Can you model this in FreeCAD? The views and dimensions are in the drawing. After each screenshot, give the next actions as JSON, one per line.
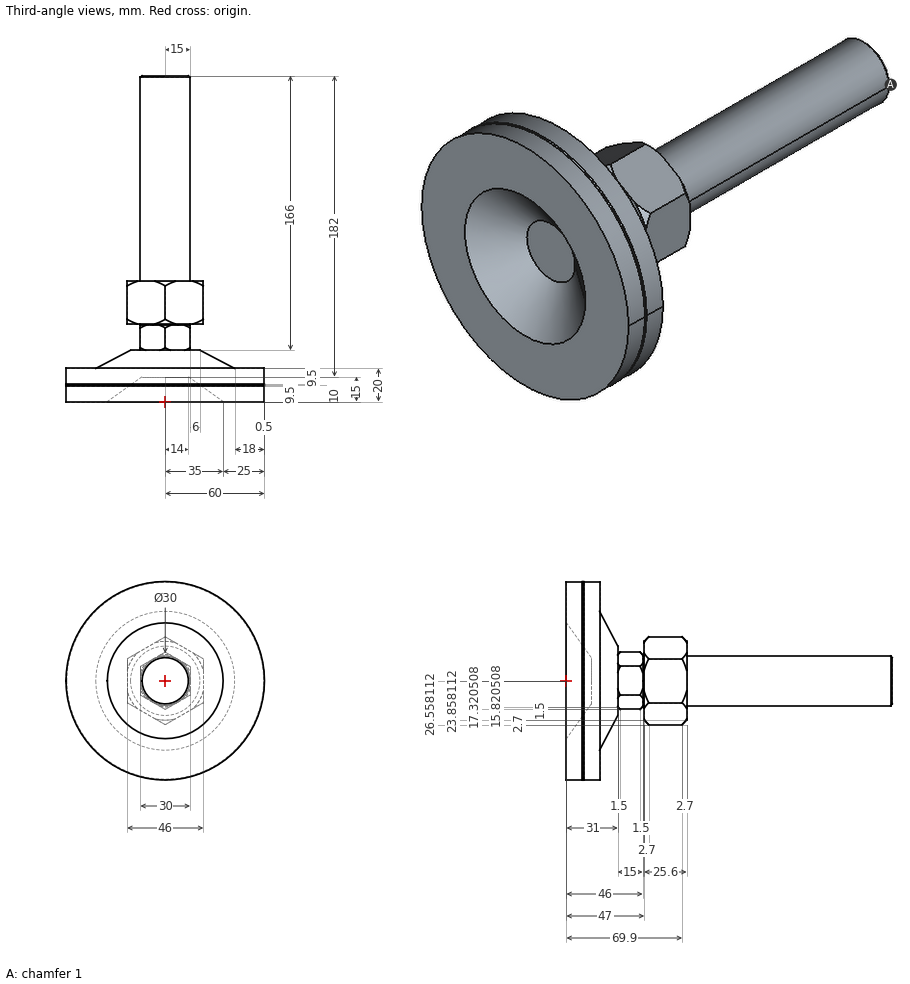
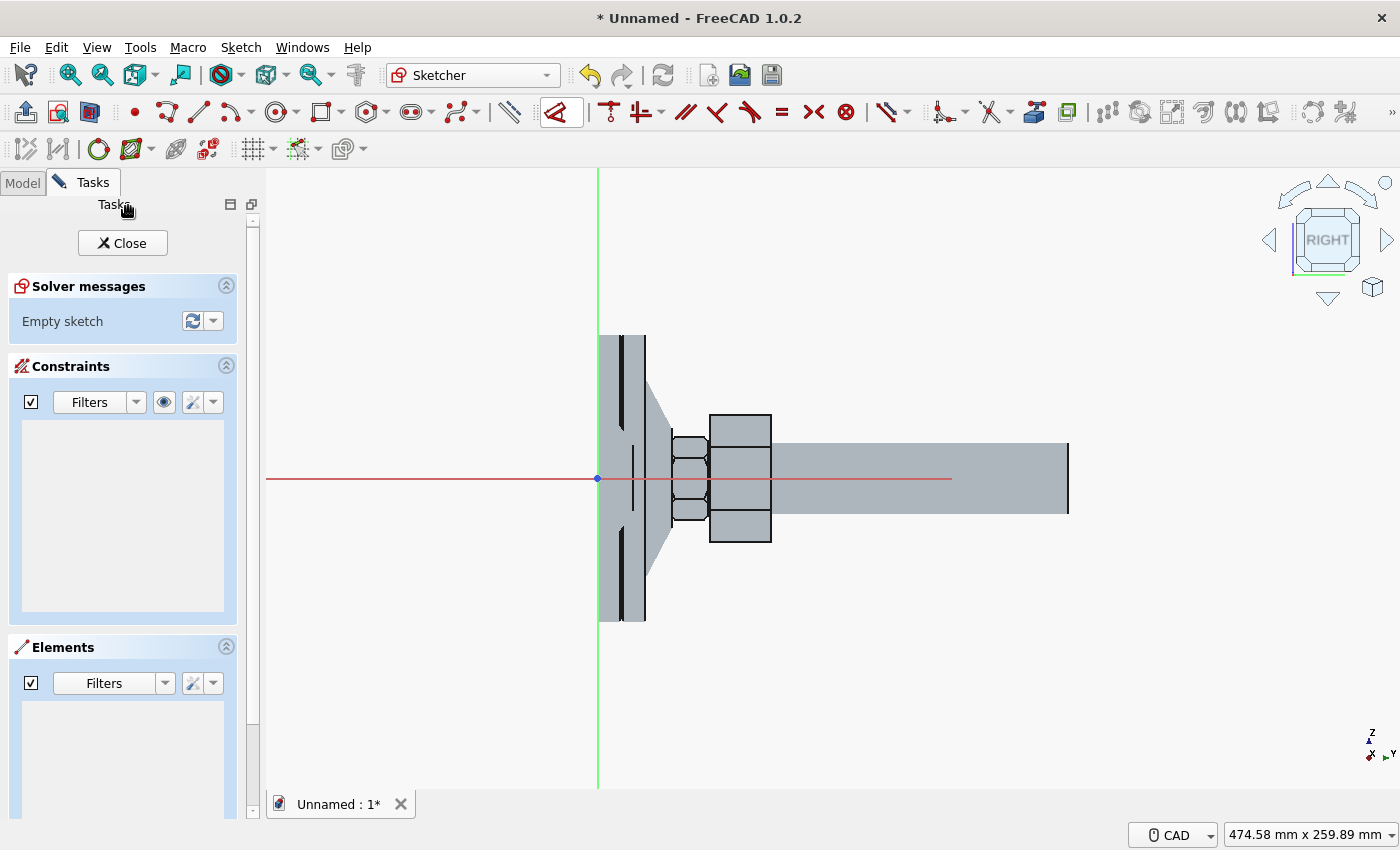
{"action": "scroll", "coordinate": [738, 545], "scroll_direction": "up", "scroll_amount": 12}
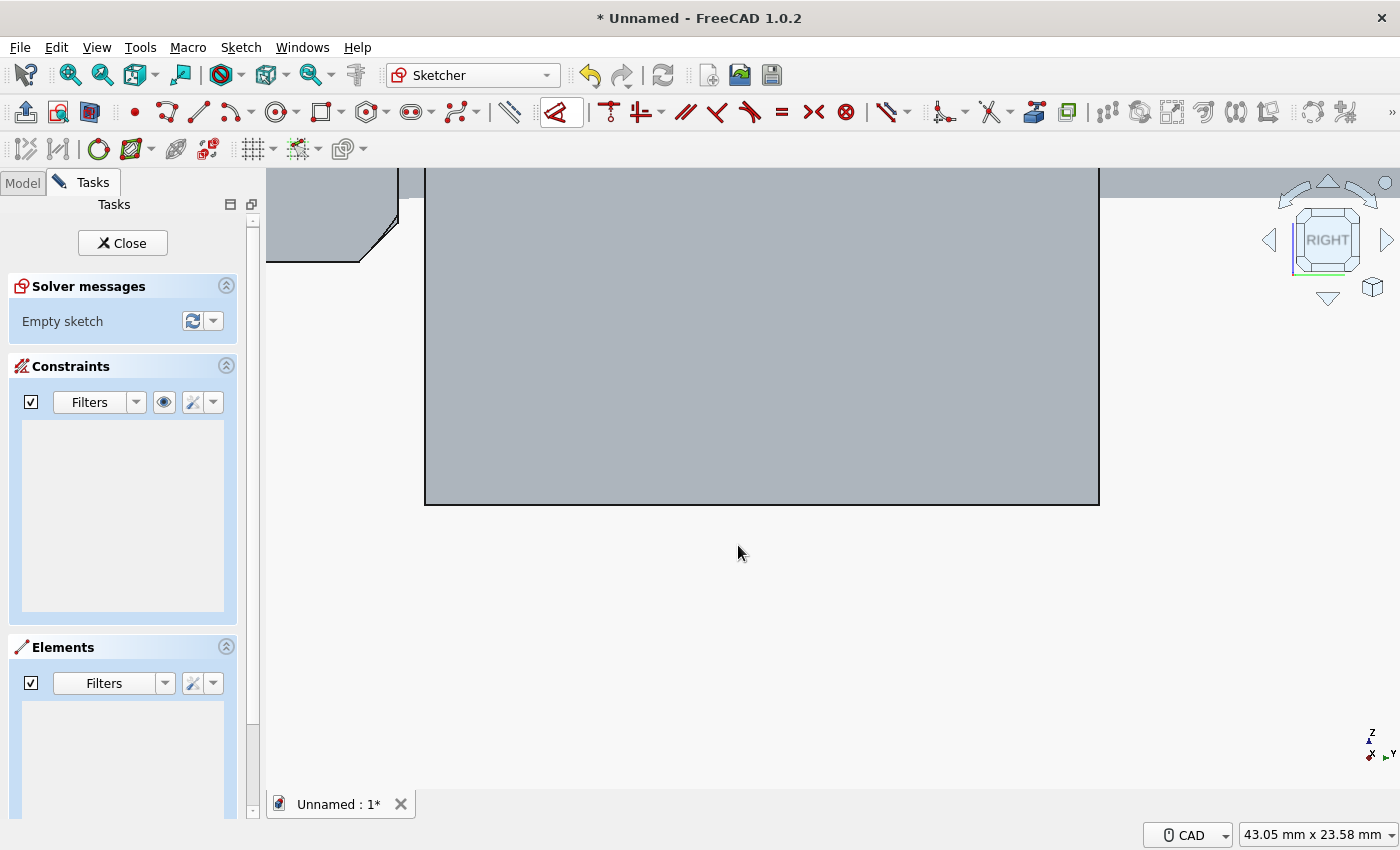
{"action": "key", "text": "g m"}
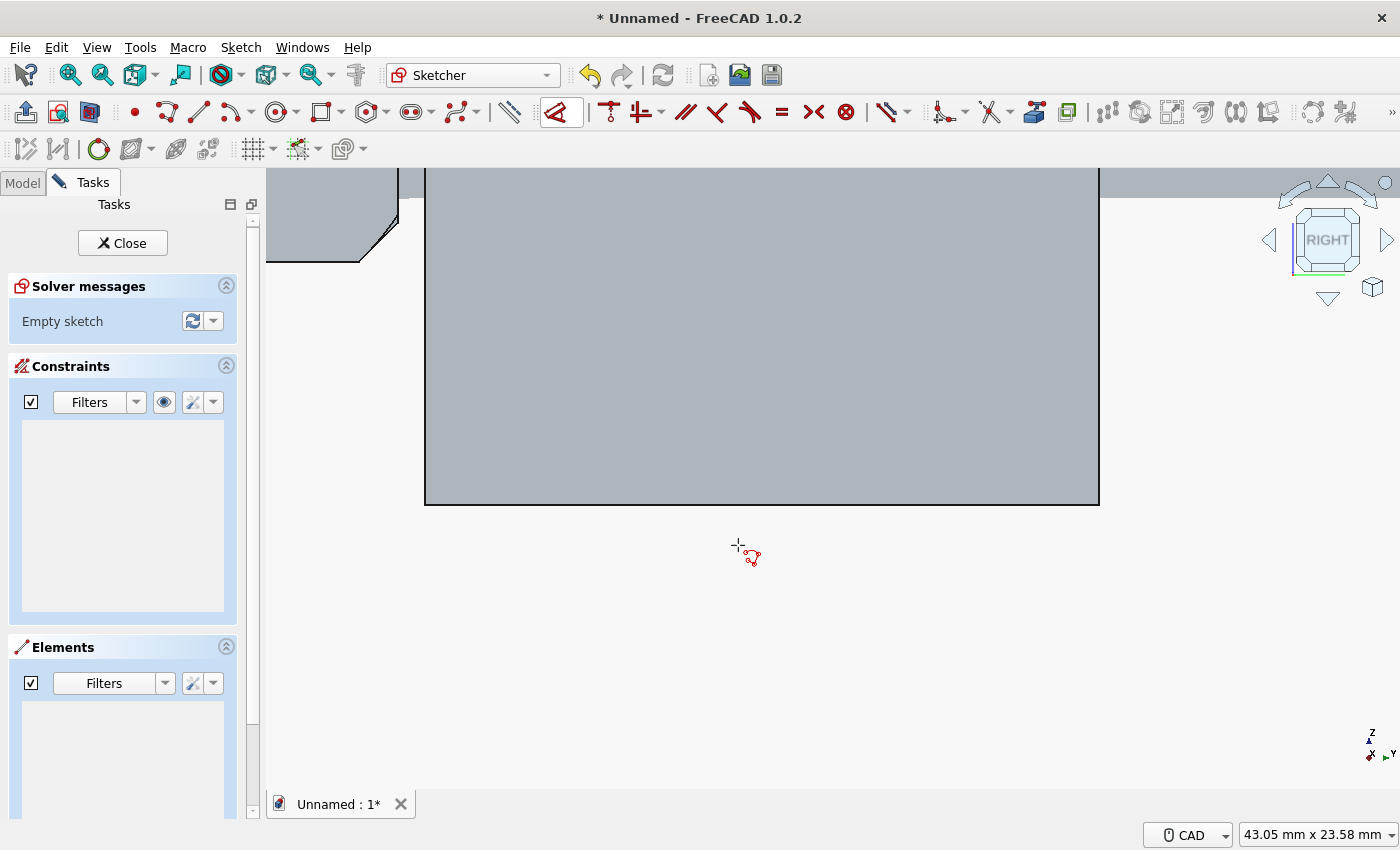
{"action": "left_click", "coordinate": [1028, 505]}
{"action": "left_click", "coordinate": [1099, 505]}
{"action": "left_click", "coordinate": [1099, 434]}
{"action": "left_click", "coordinate": [1028, 506]}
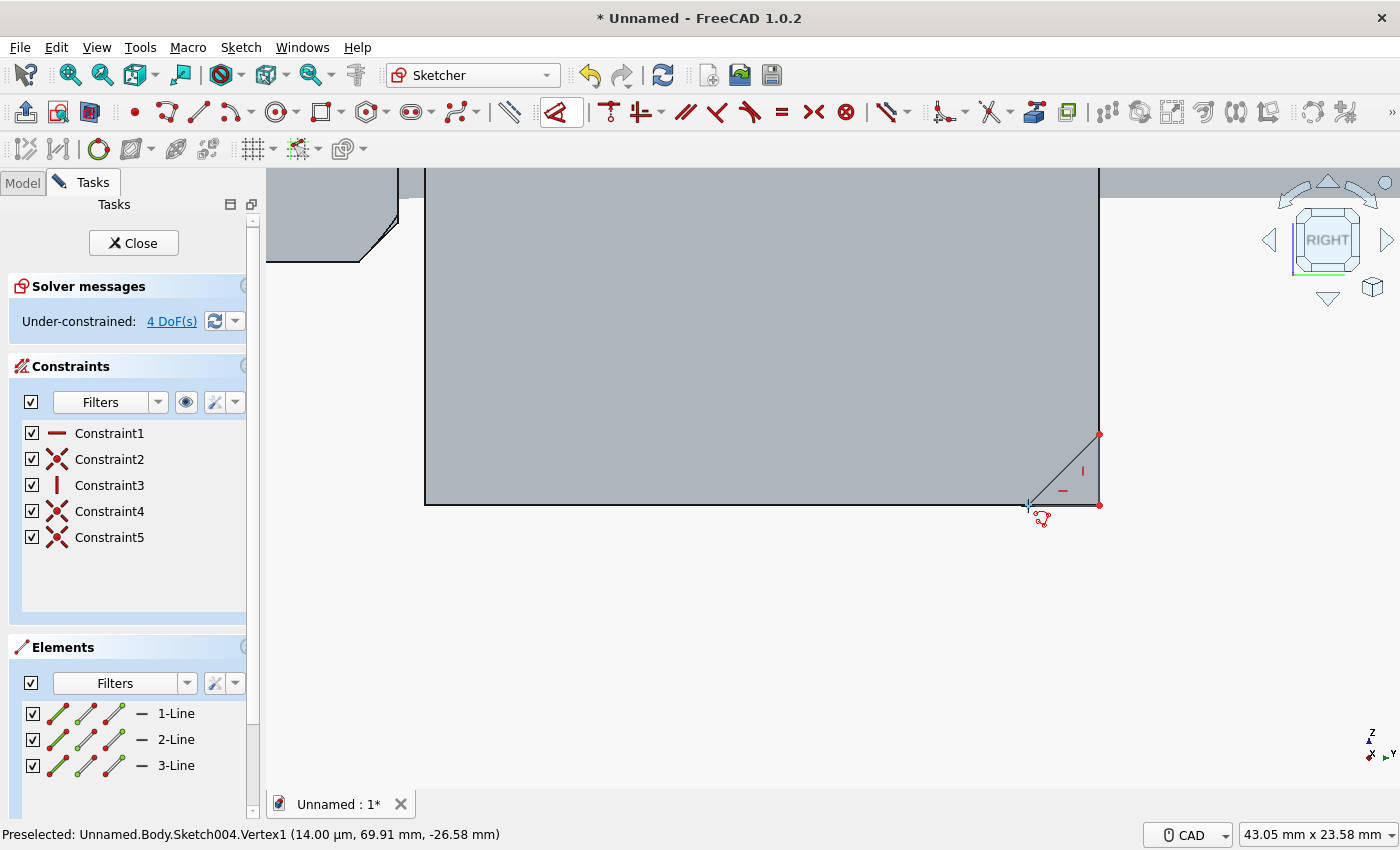
{"action": "left_click", "coordinate": [425, 434]}
{"action": "left_click", "coordinate": [425, 505]}
{"action": "left_click", "coordinate": [496, 505]}
{"action": "left_click", "coordinate": [425, 435]}
{"action": "key", "text": "Escape"}
{"action": "key", "text": "Escape"}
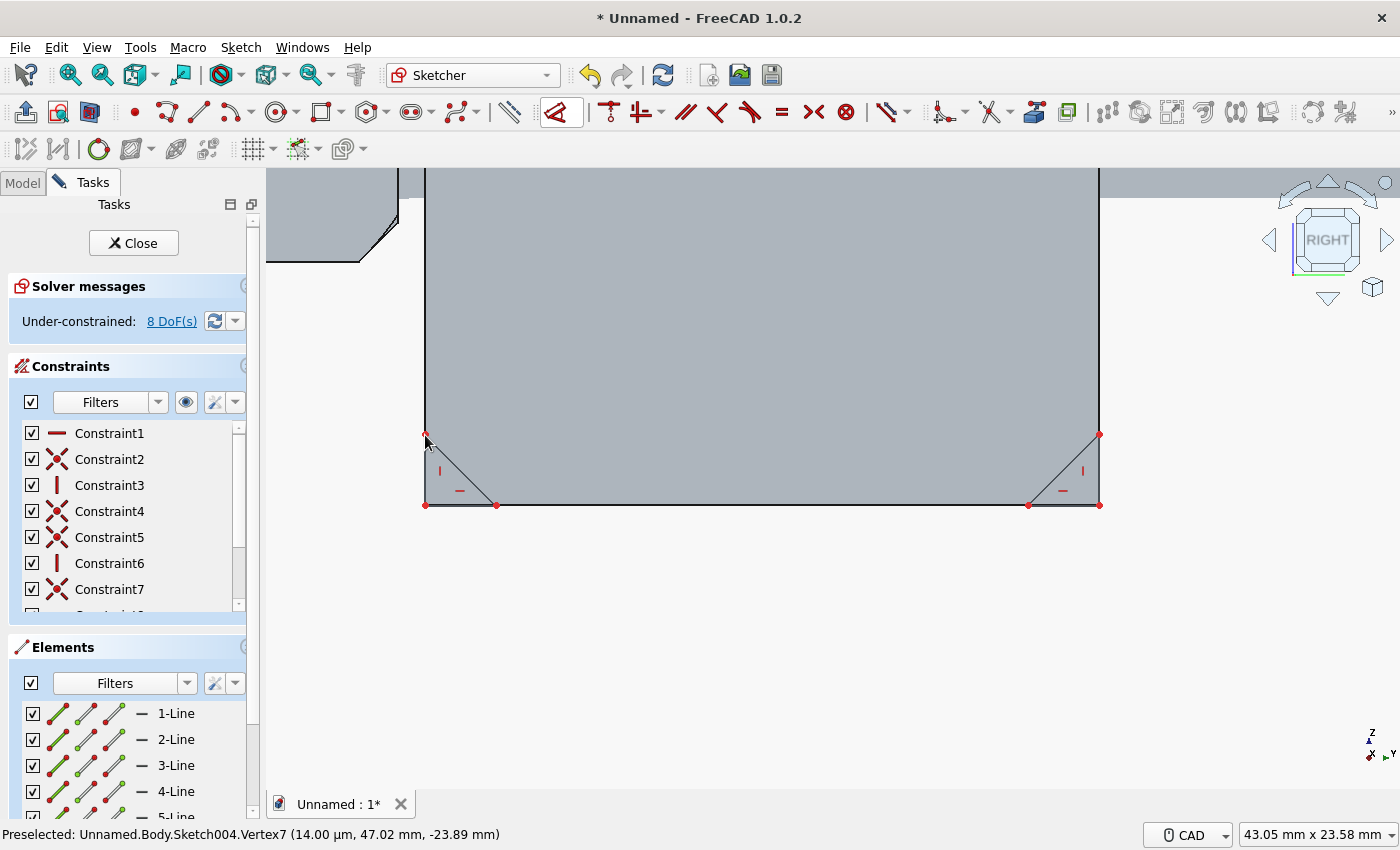
{"action": "left_click", "coordinate": [1049, 506]}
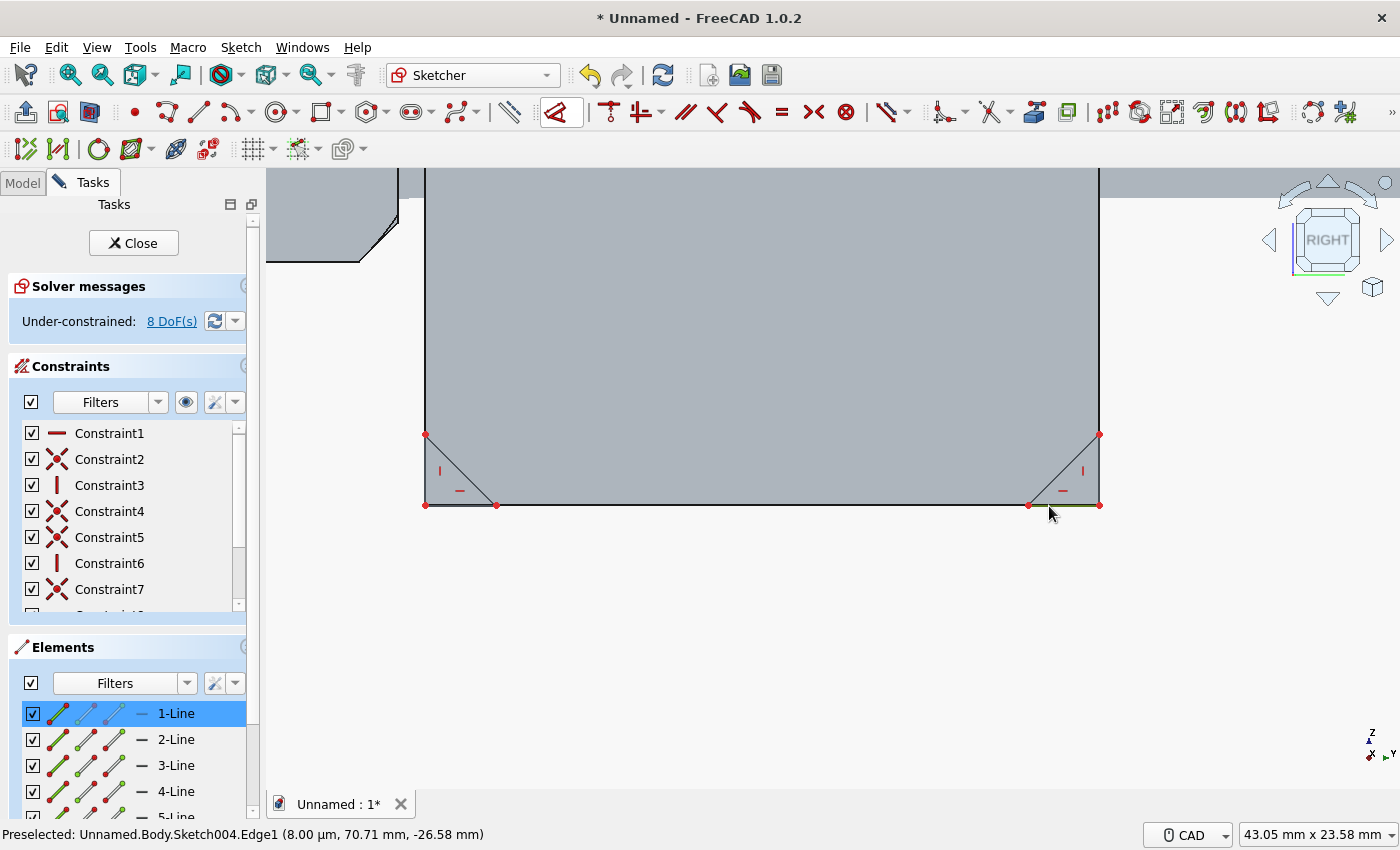
{"action": "key", "text": "l"}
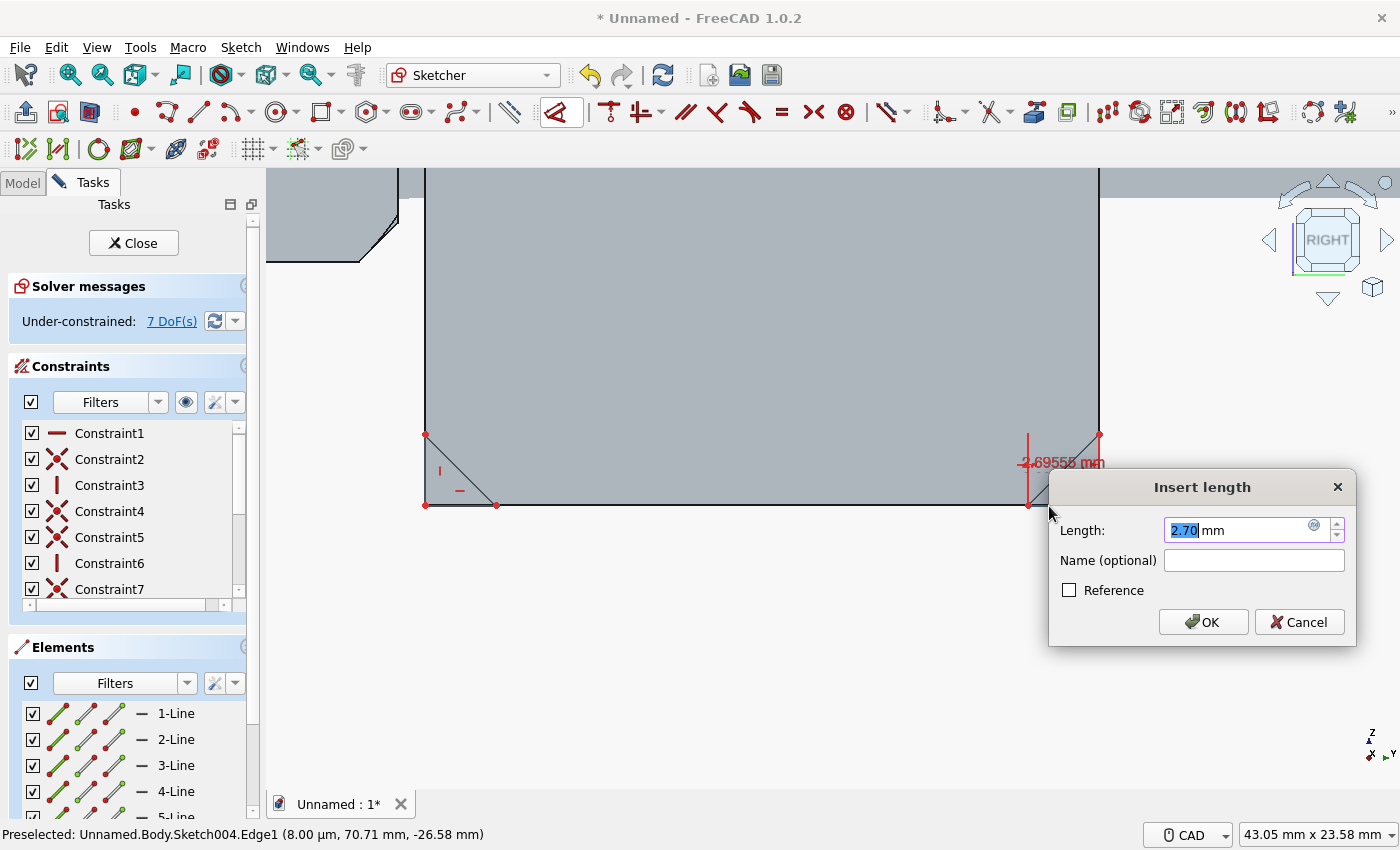
{"action": "type", "text": "2.7"}
{"action": "key", "text": "Return"}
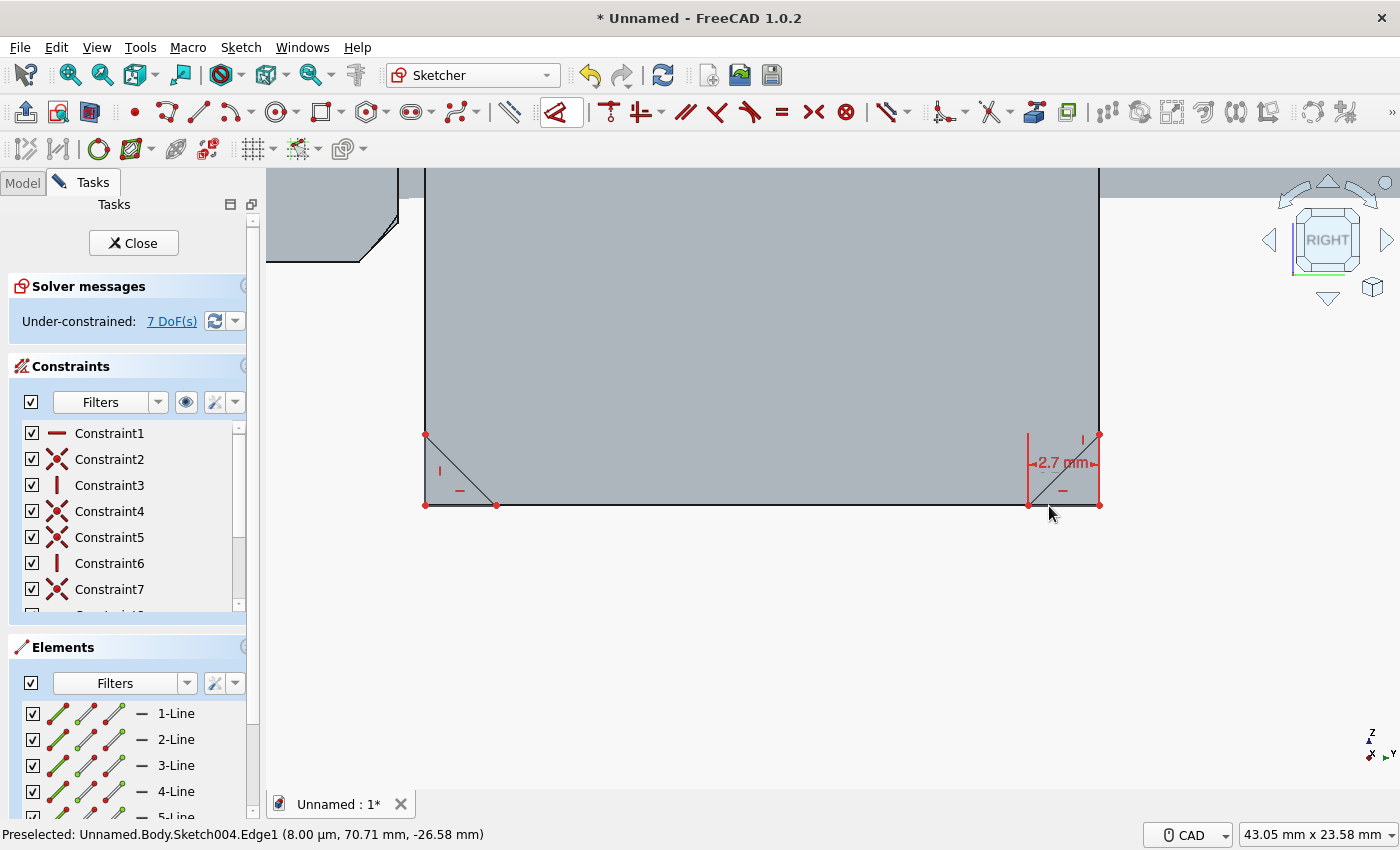
{"action": "left_click", "coordinate": [1099, 485]}